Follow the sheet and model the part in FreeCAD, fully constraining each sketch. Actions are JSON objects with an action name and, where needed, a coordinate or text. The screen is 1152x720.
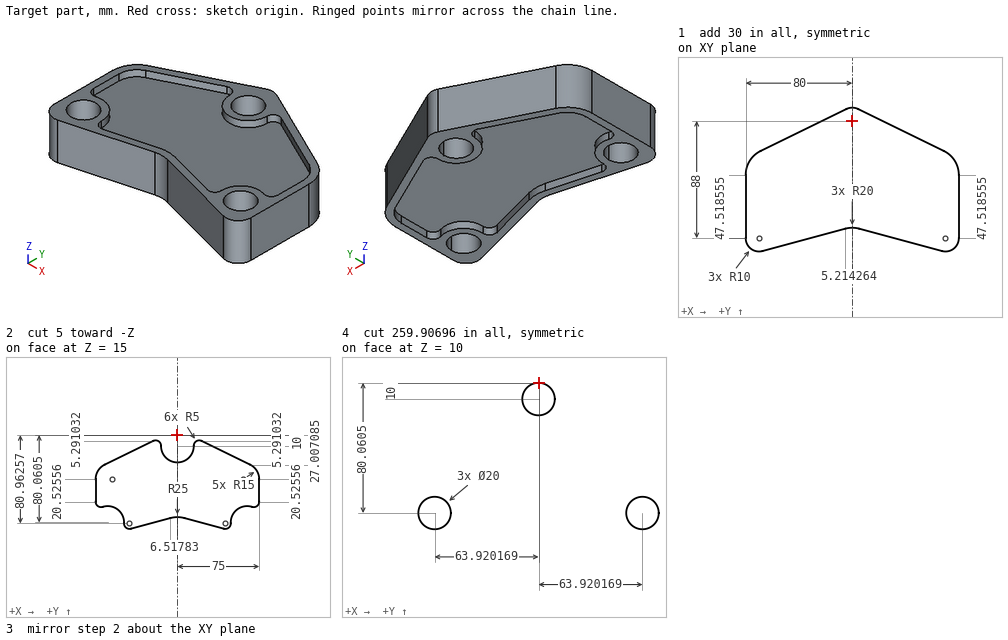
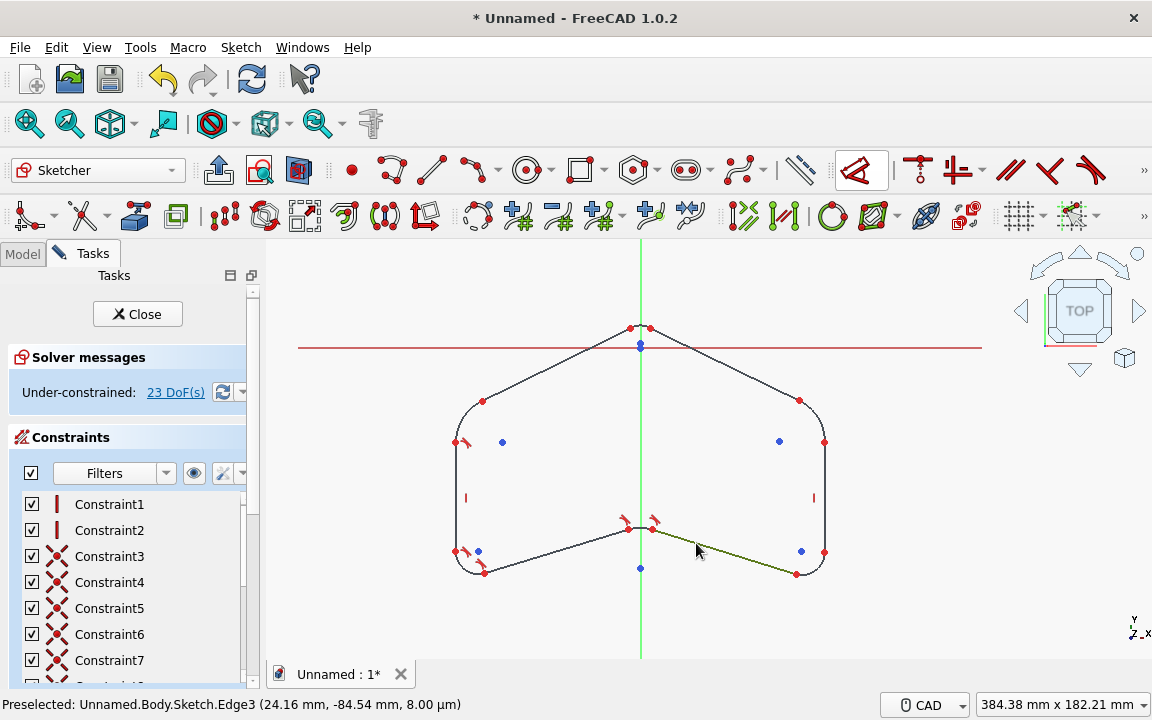
{"action": "left_click", "coordinate": [808, 574]}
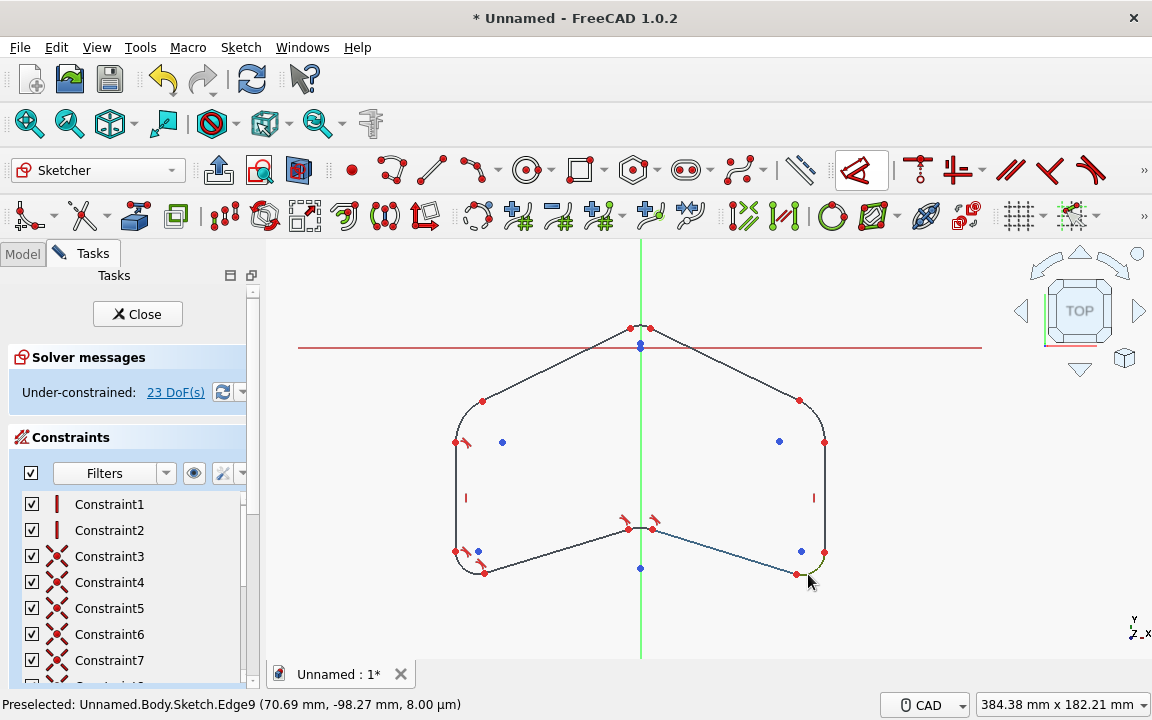
{"action": "key", "text": "t"}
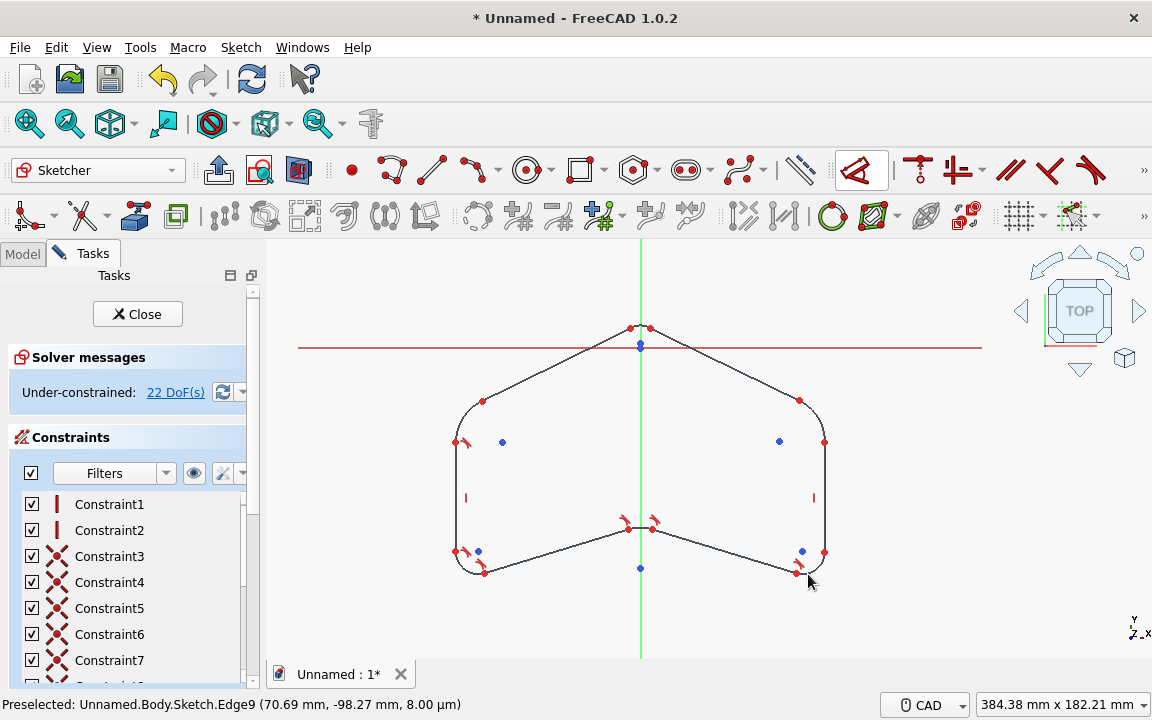
{"action": "left_click", "coordinate": [825, 519]}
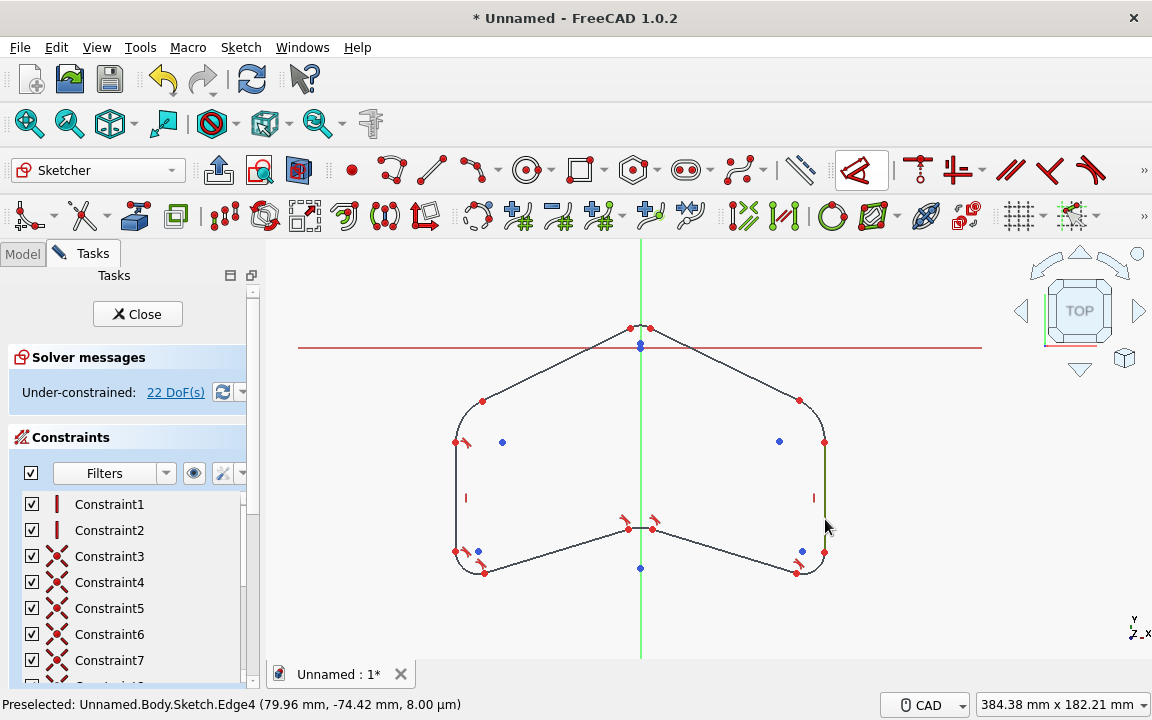
{"action": "left_click", "coordinate": [808, 573]}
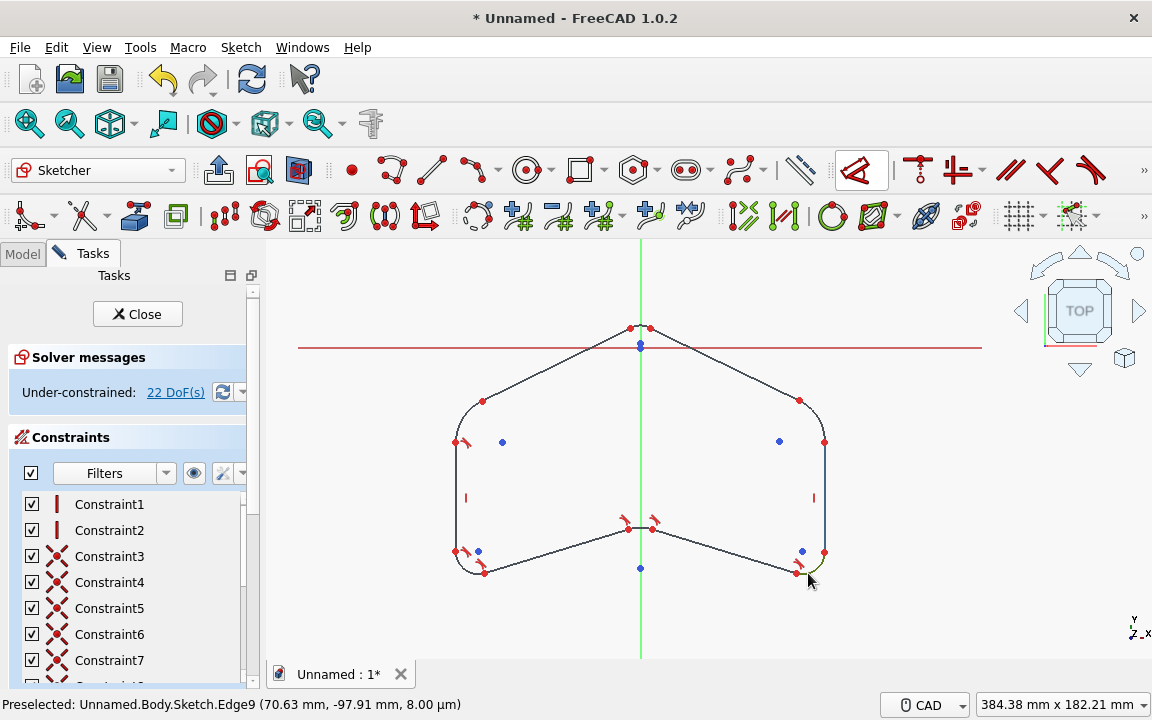
{"action": "left_click", "coordinate": [1092, 170]}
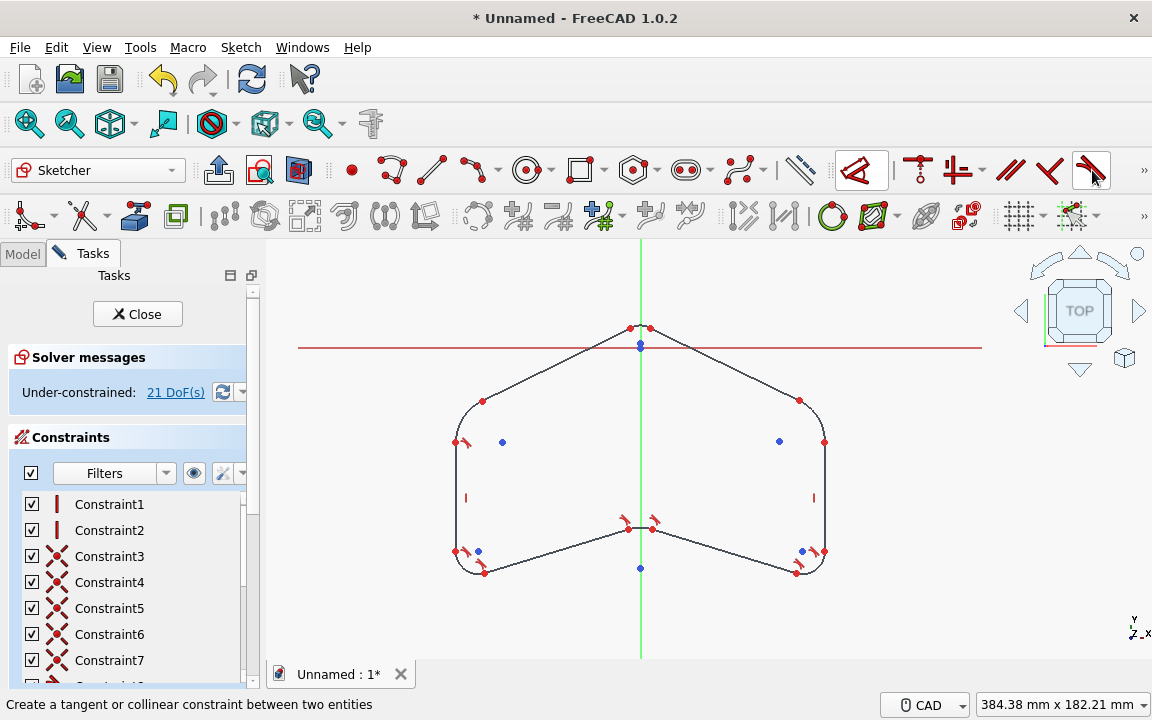
{"action": "left_click", "coordinate": [825, 519]}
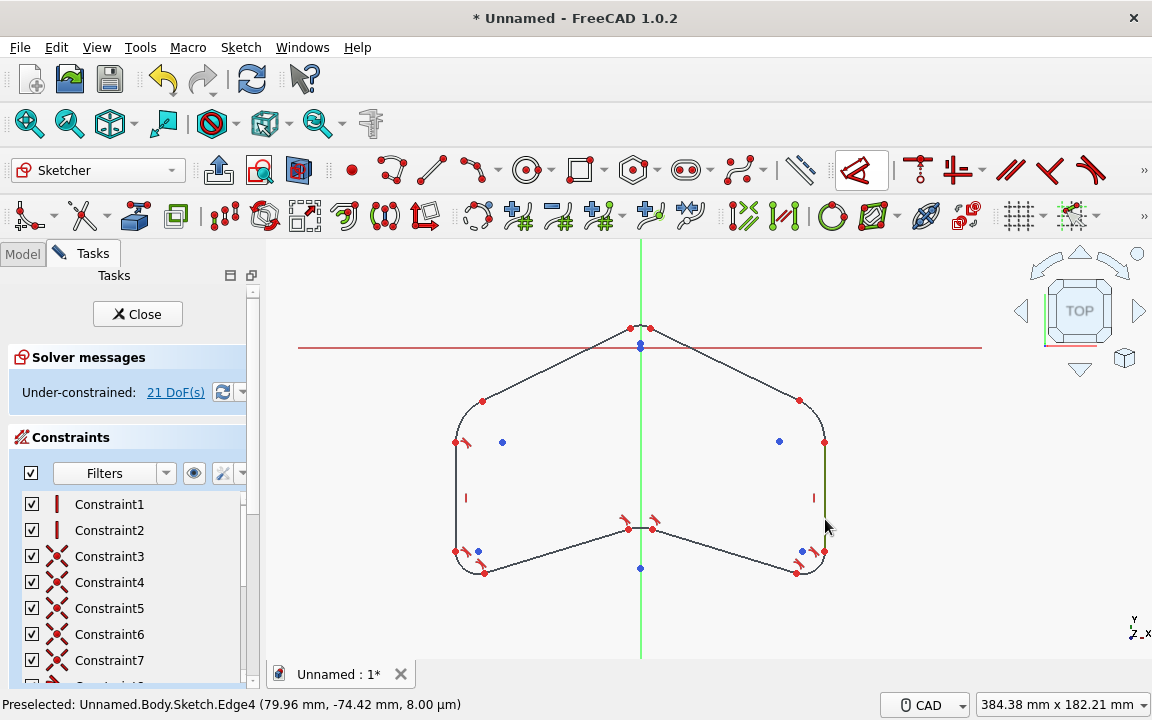
{"action": "left_click", "coordinate": [822, 427]}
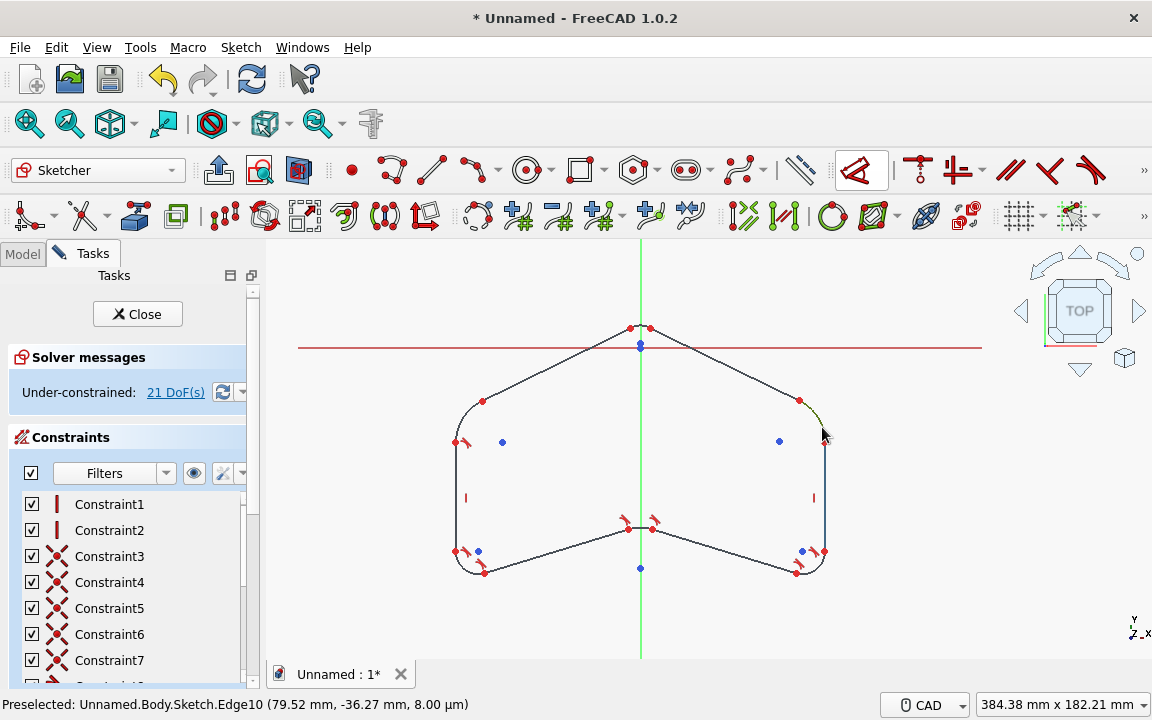
{"action": "left_click", "coordinate": [1092, 170]}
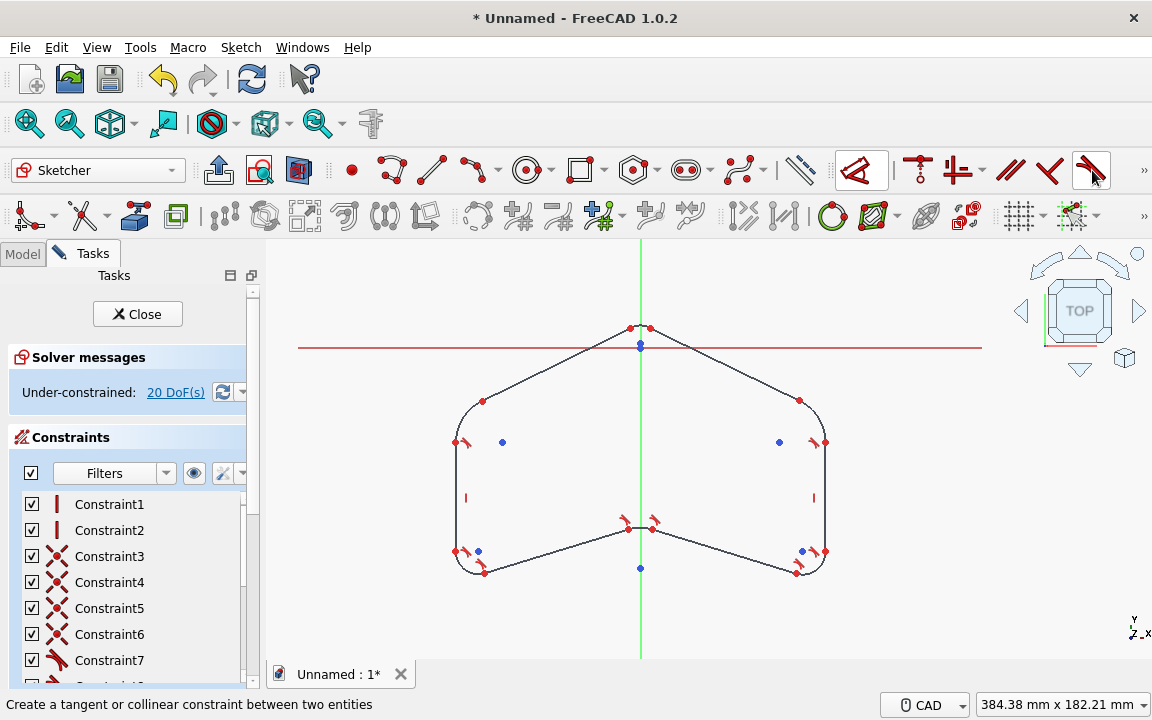
{"action": "left_click", "coordinate": [755, 379]}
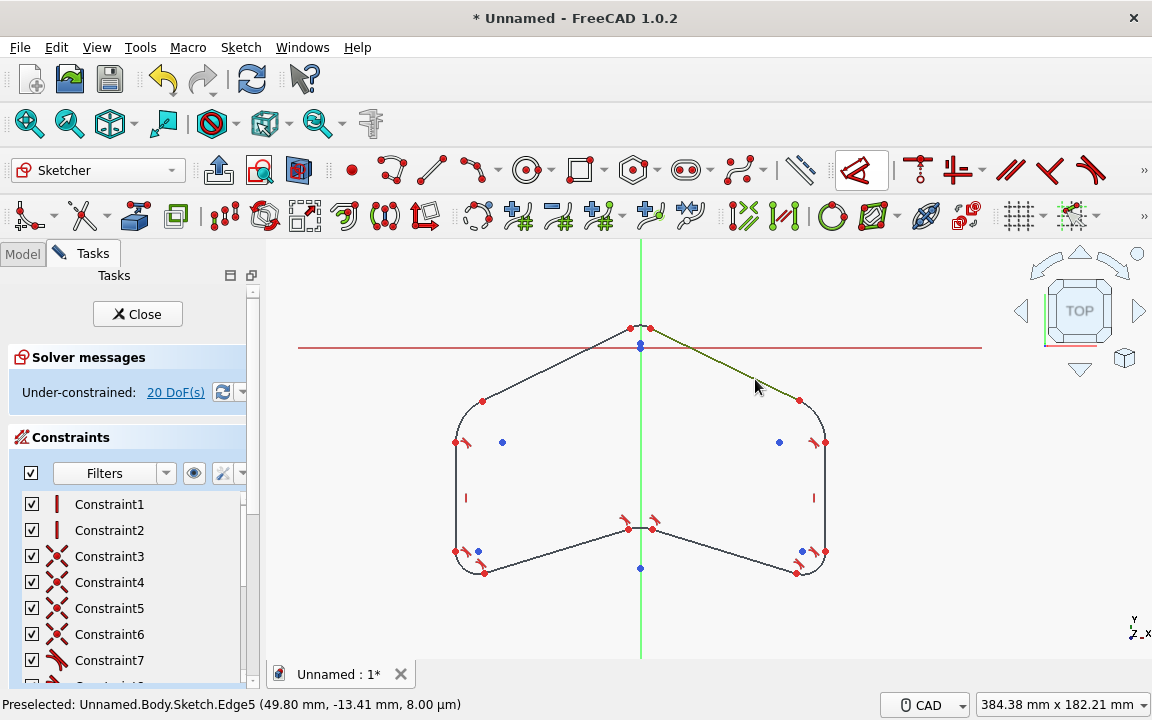
{"action": "left_click", "coordinate": [823, 427]}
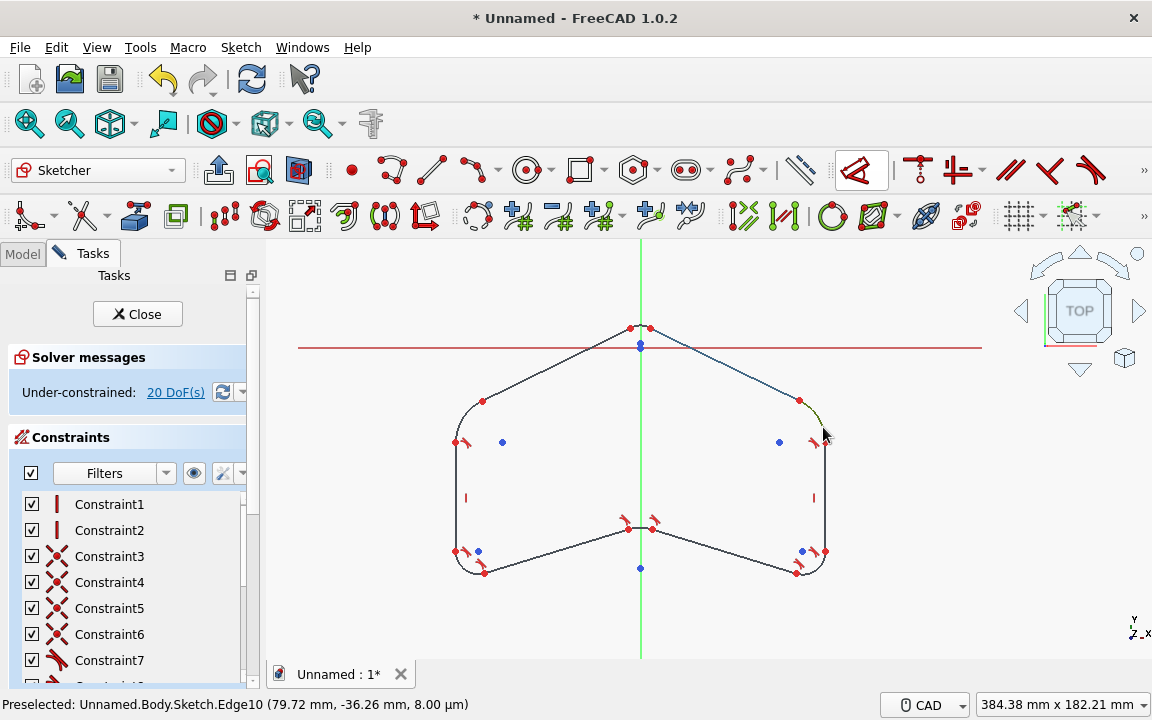
{"action": "left_click", "coordinate": [1092, 170]}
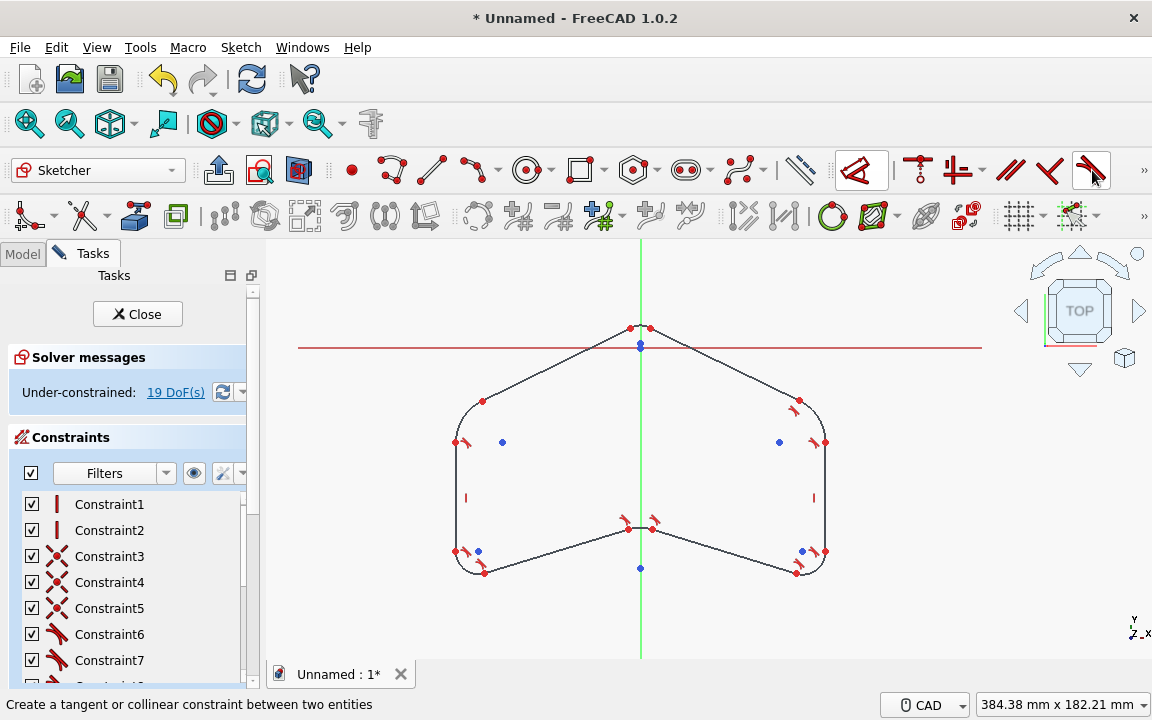
{"action": "left_click", "coordinate": [755, 379]}